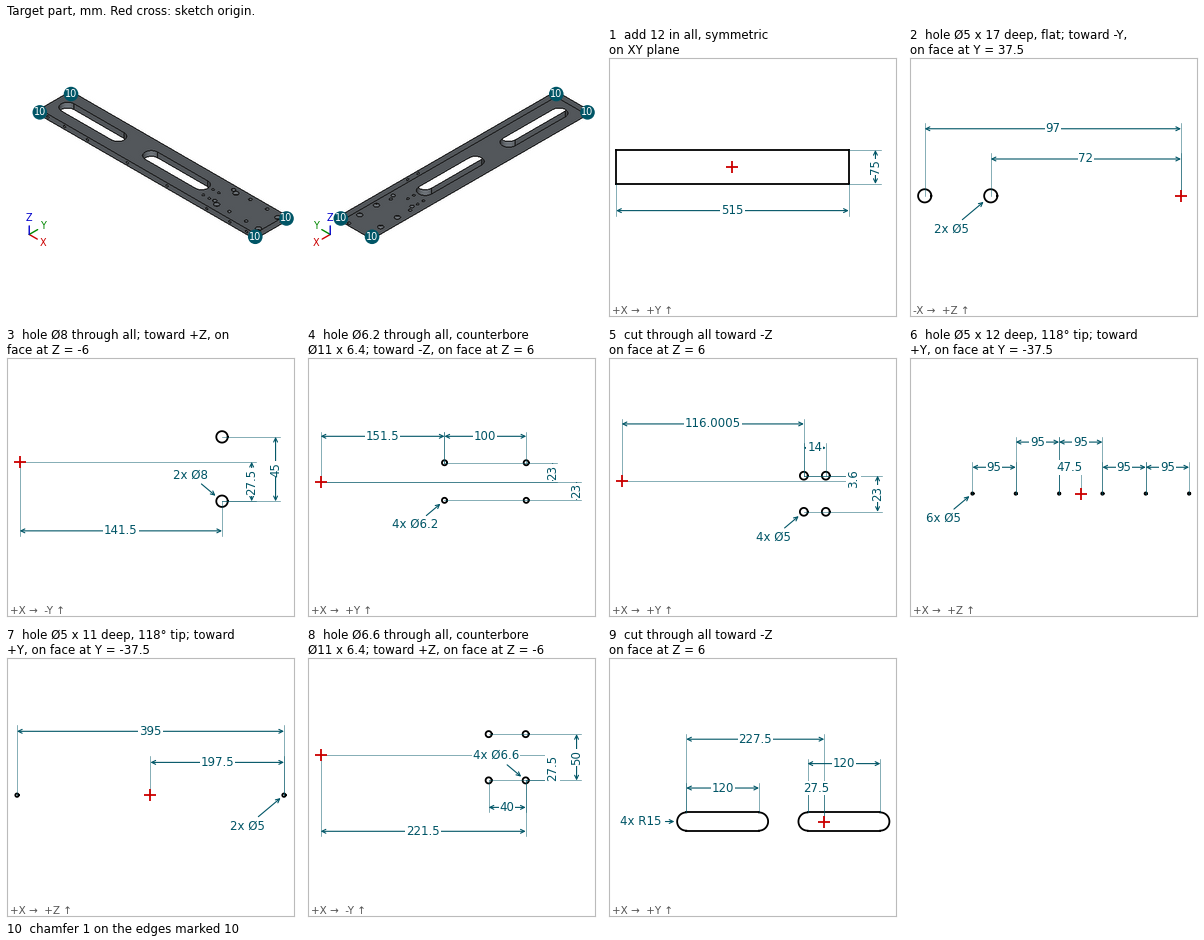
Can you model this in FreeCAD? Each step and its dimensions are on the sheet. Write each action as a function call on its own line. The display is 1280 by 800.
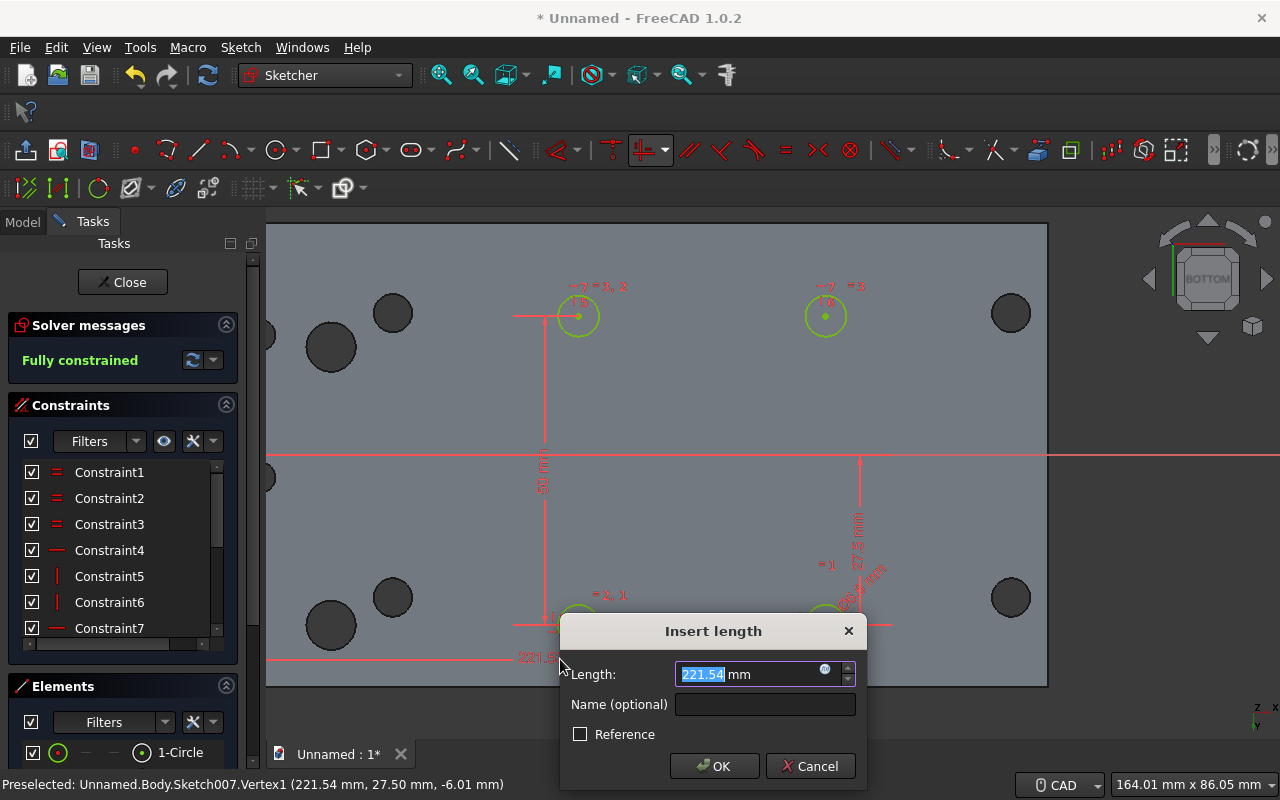
text(221.5)
key(Return)
key(Escape)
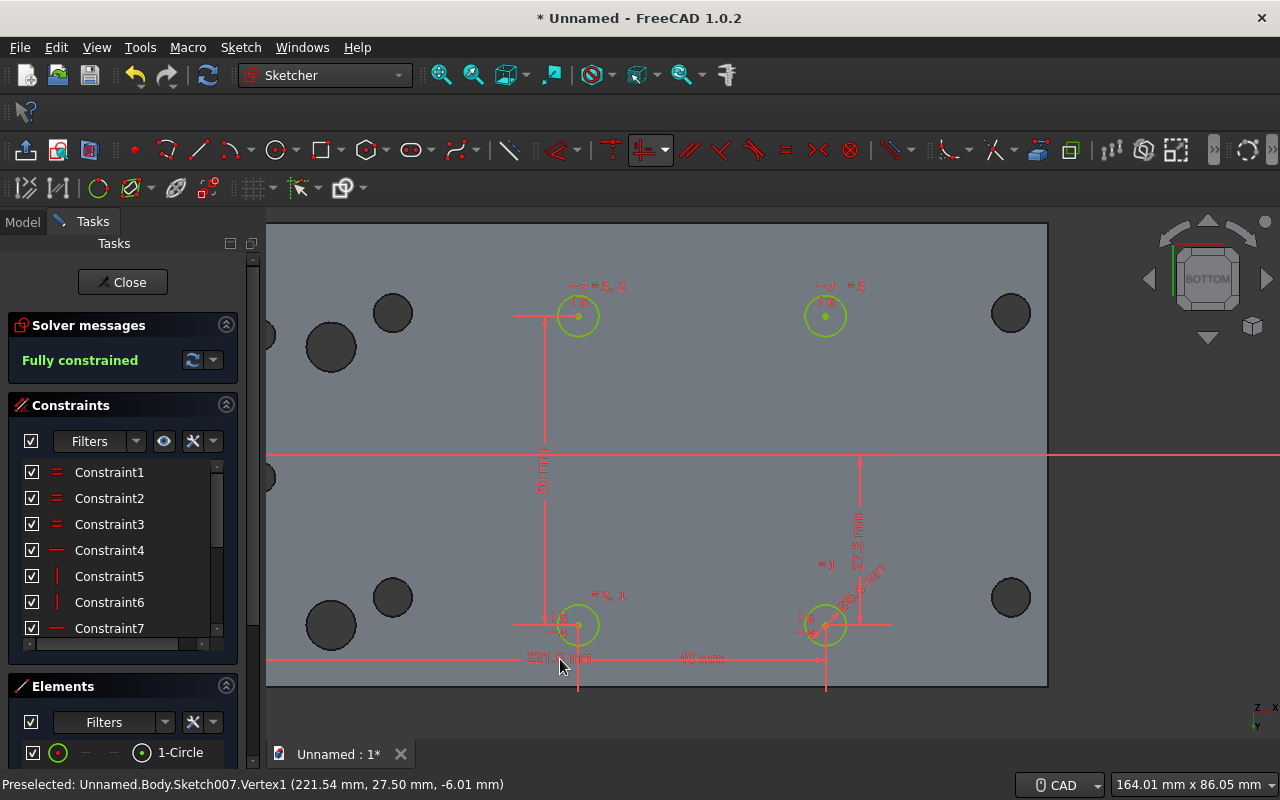
click(123, 282)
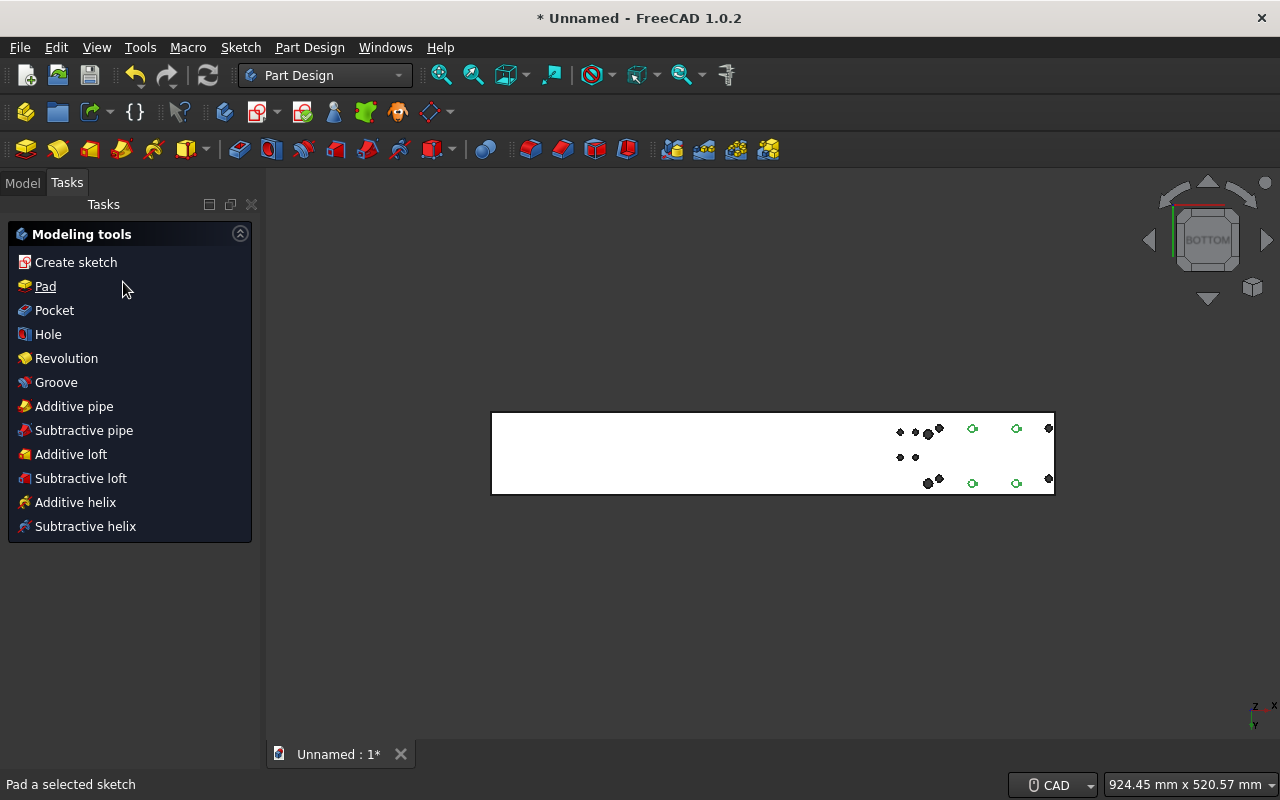
click(272, 150)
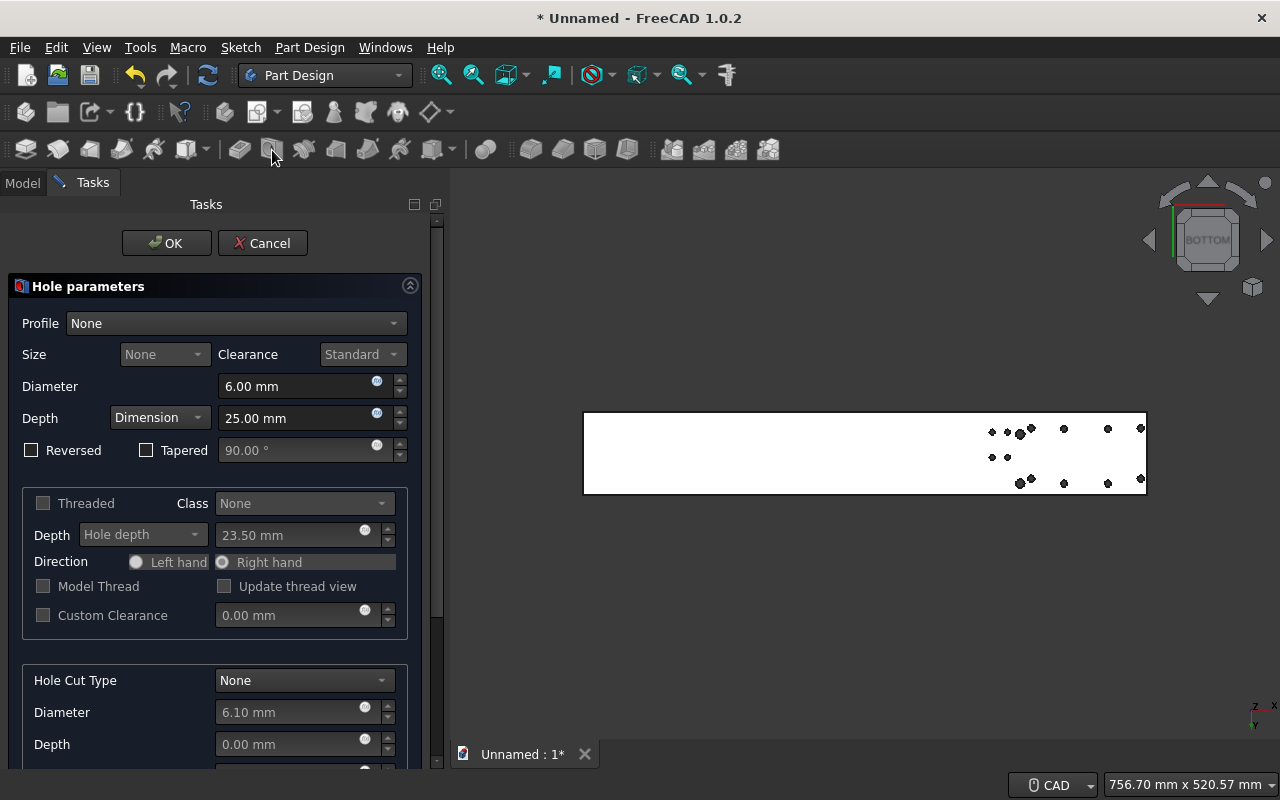
triple_click(305, 386)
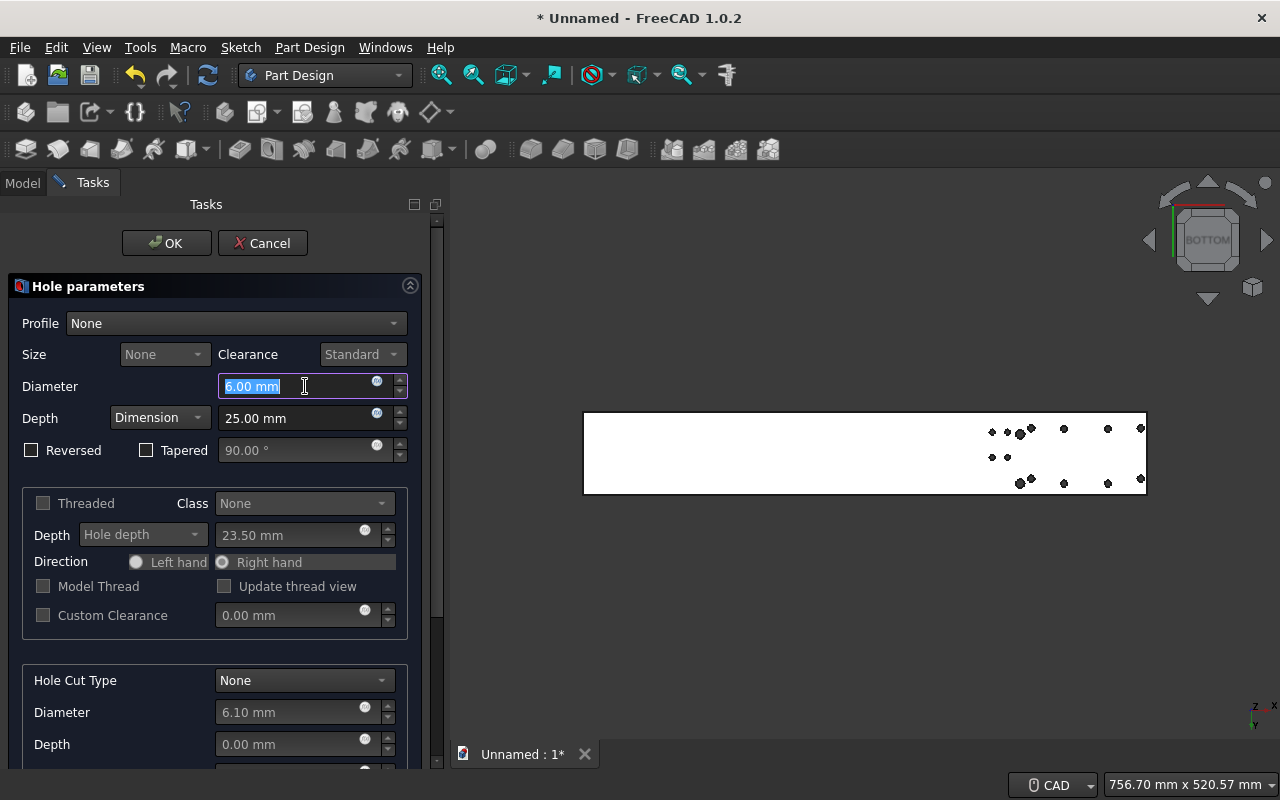
text(6.6)
key(Tab)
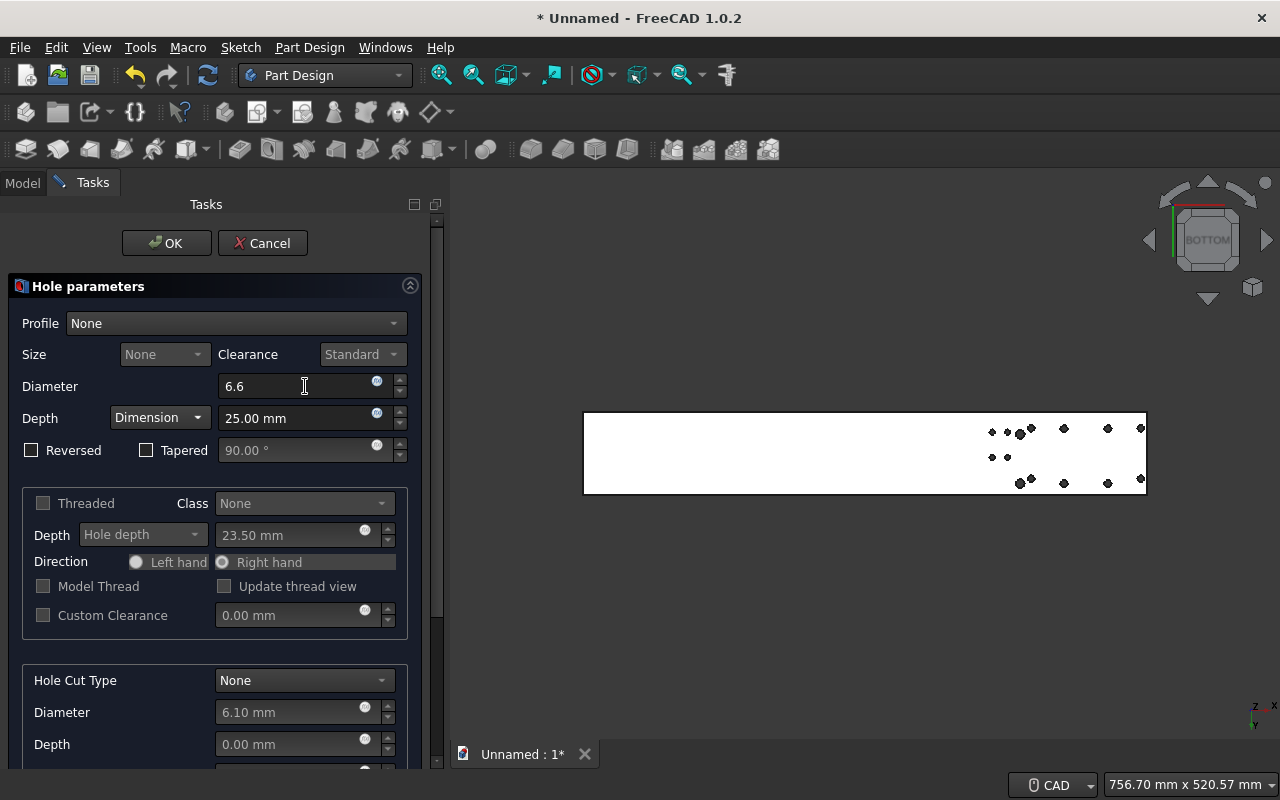
click(161, 418)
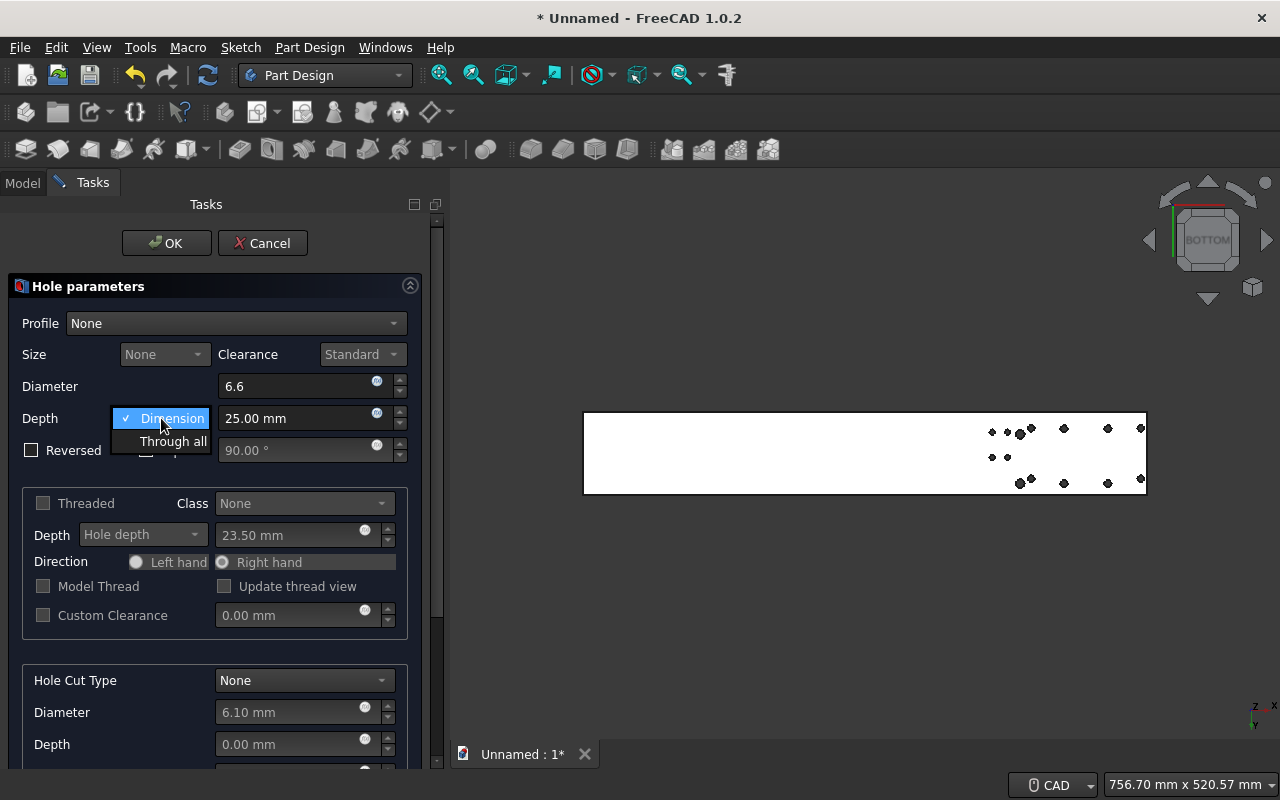
click(160, 442)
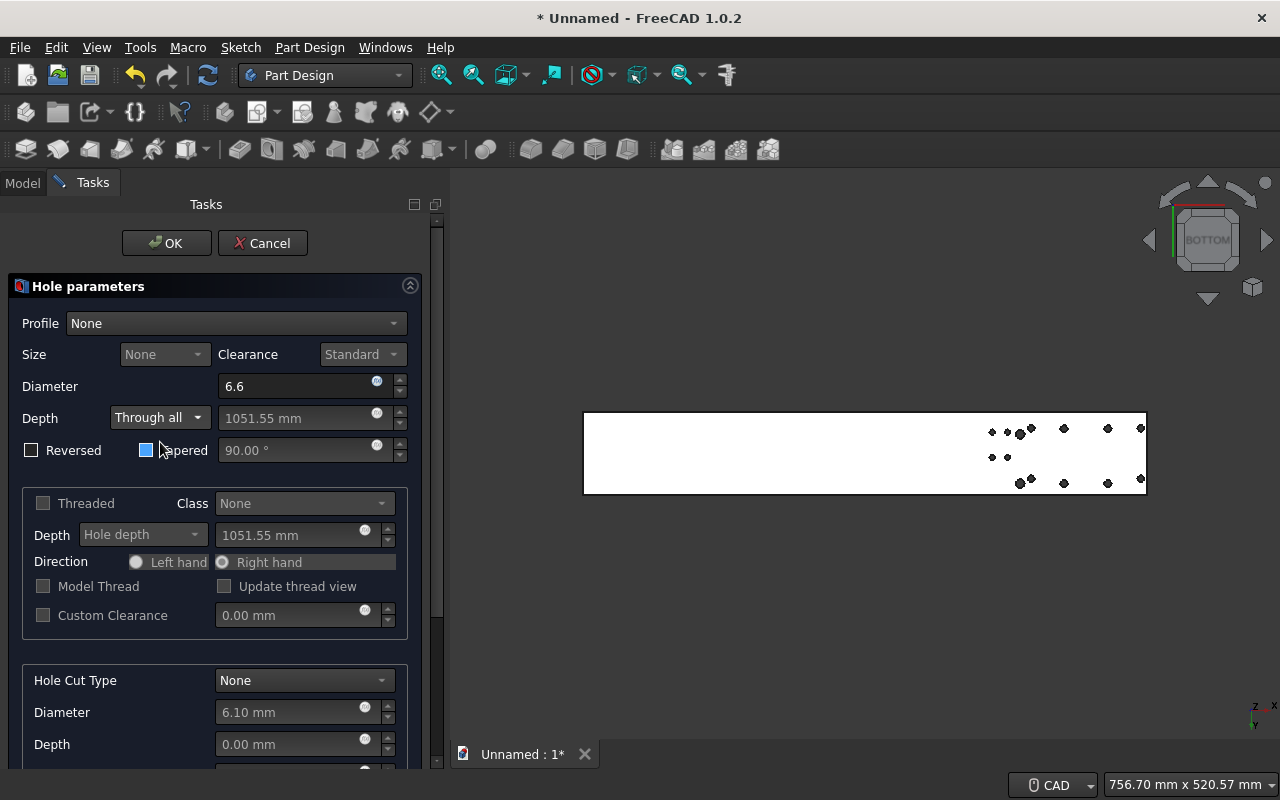
click(306, 680)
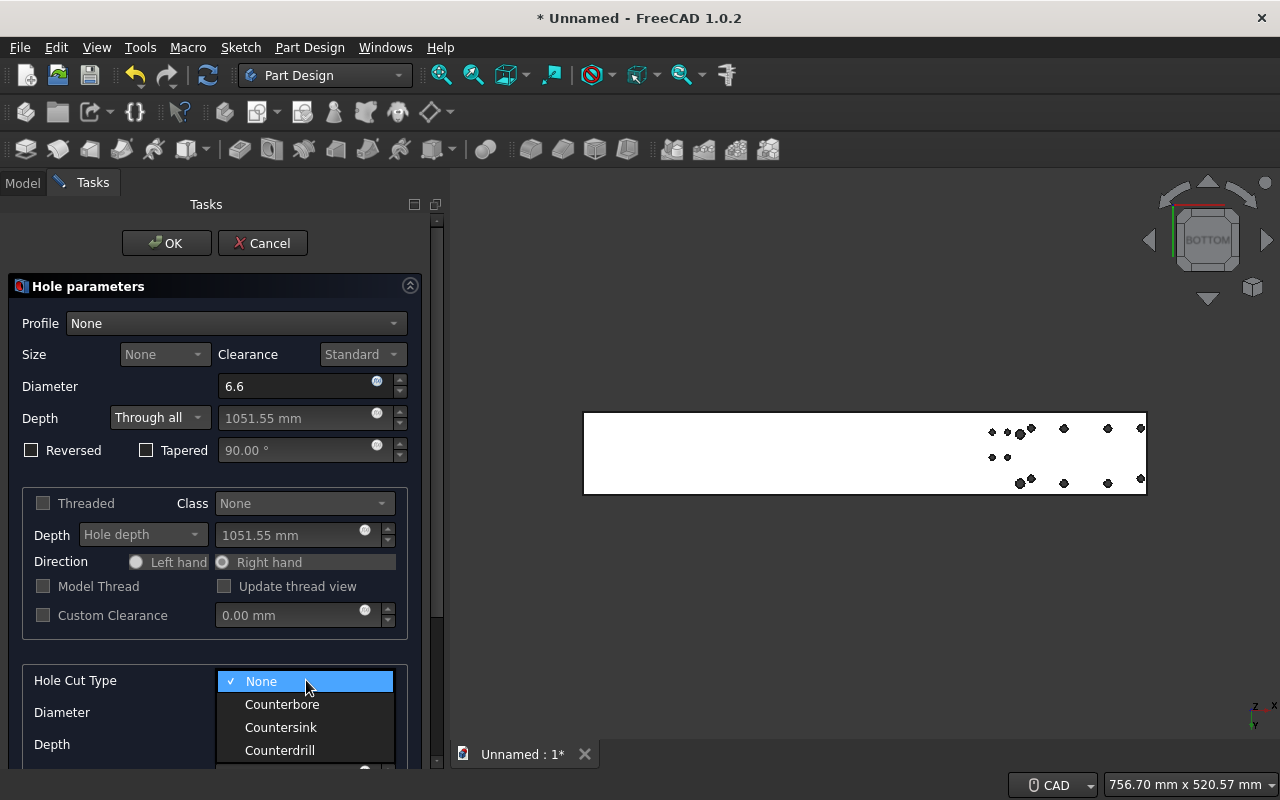
click(304, 704)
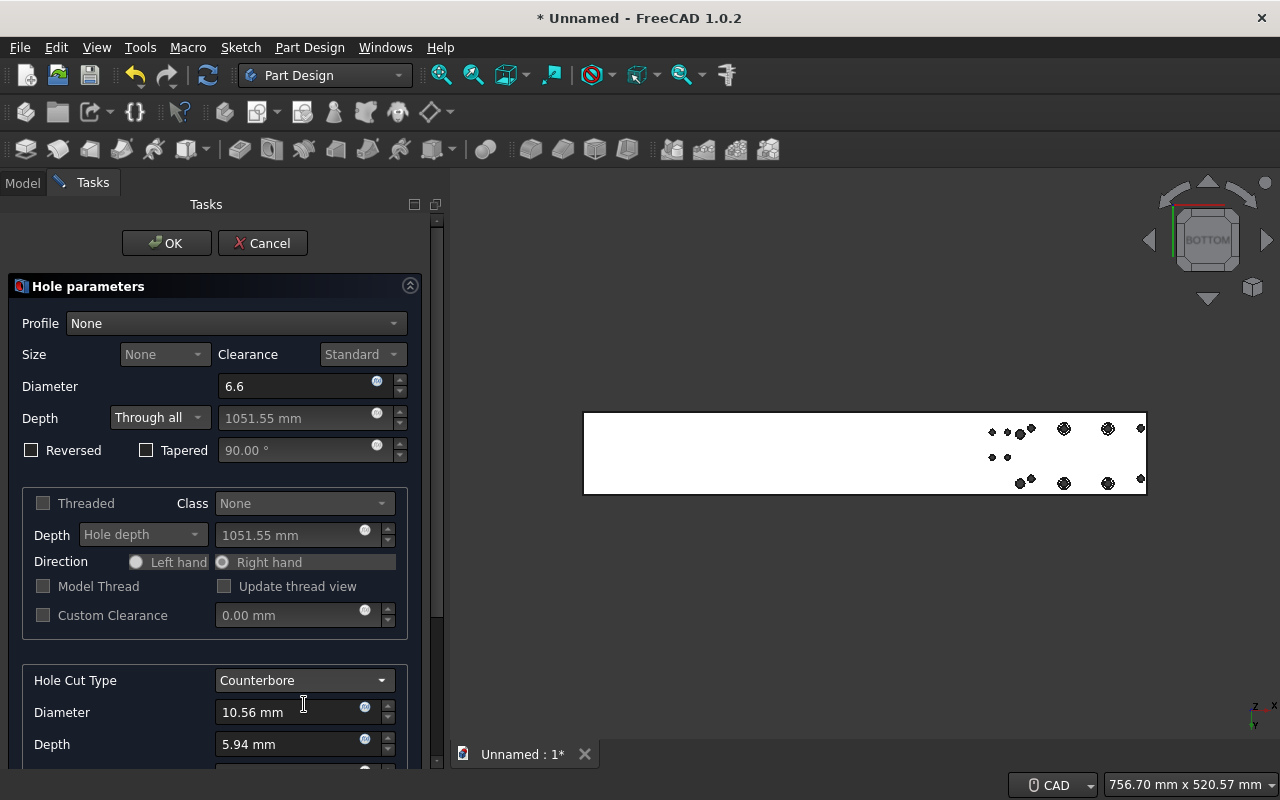
triple_click(298, 712)